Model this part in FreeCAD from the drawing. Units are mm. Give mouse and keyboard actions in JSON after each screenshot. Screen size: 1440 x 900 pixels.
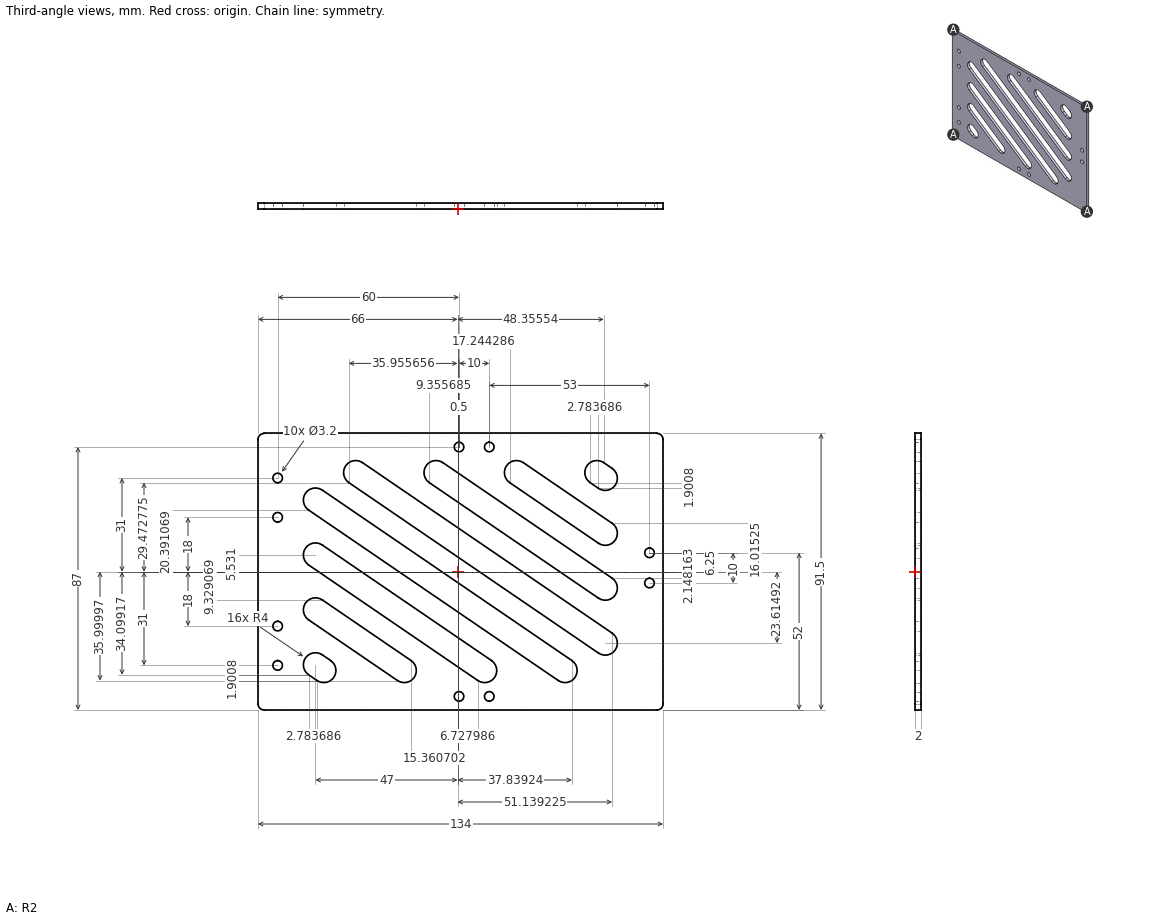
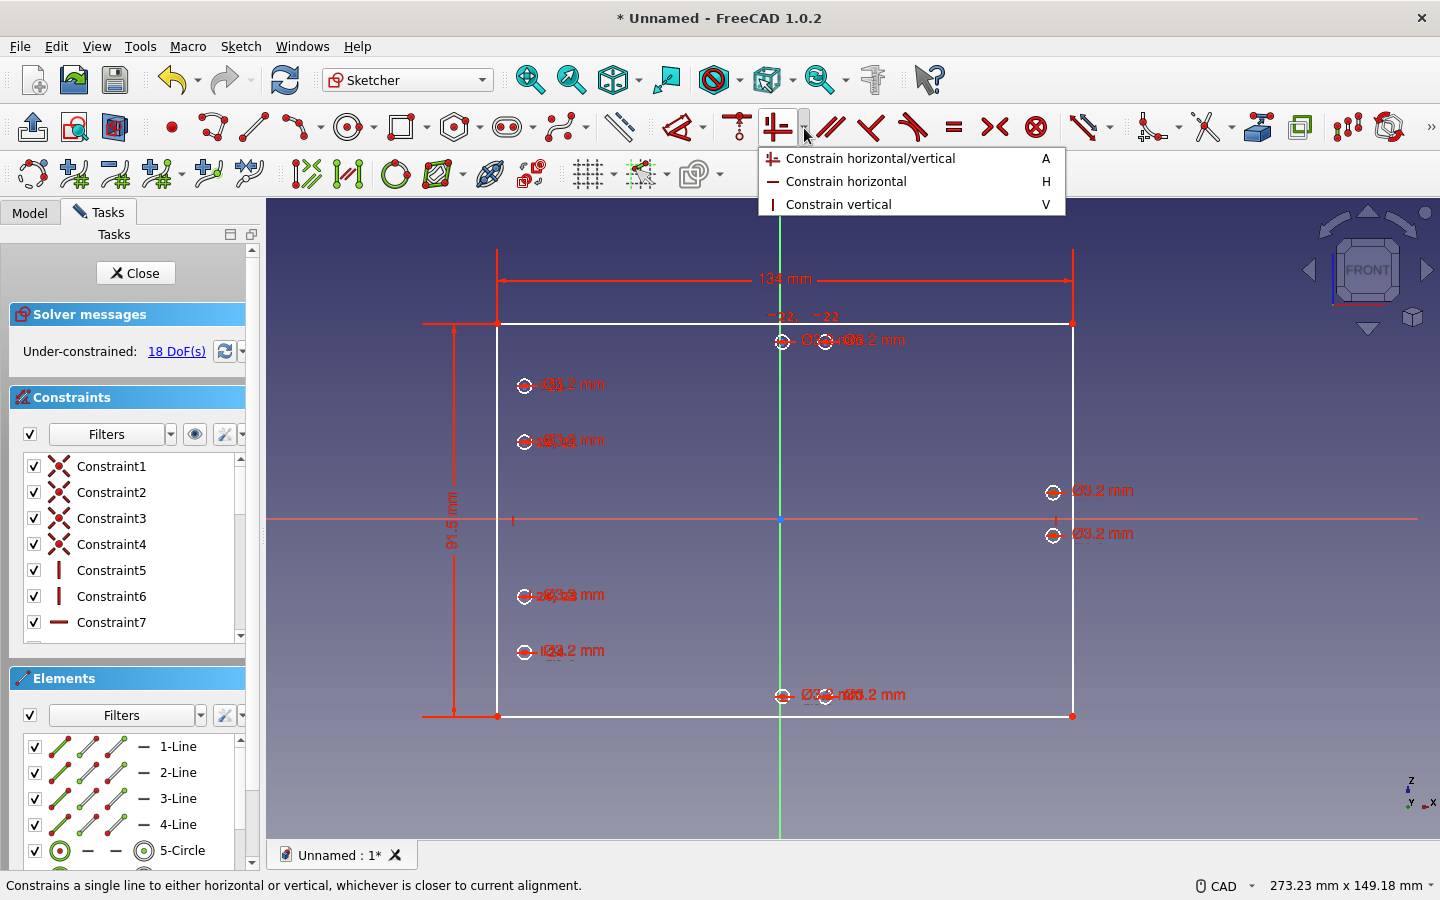
{"action": "left_click", "coordinate": [912, 204]}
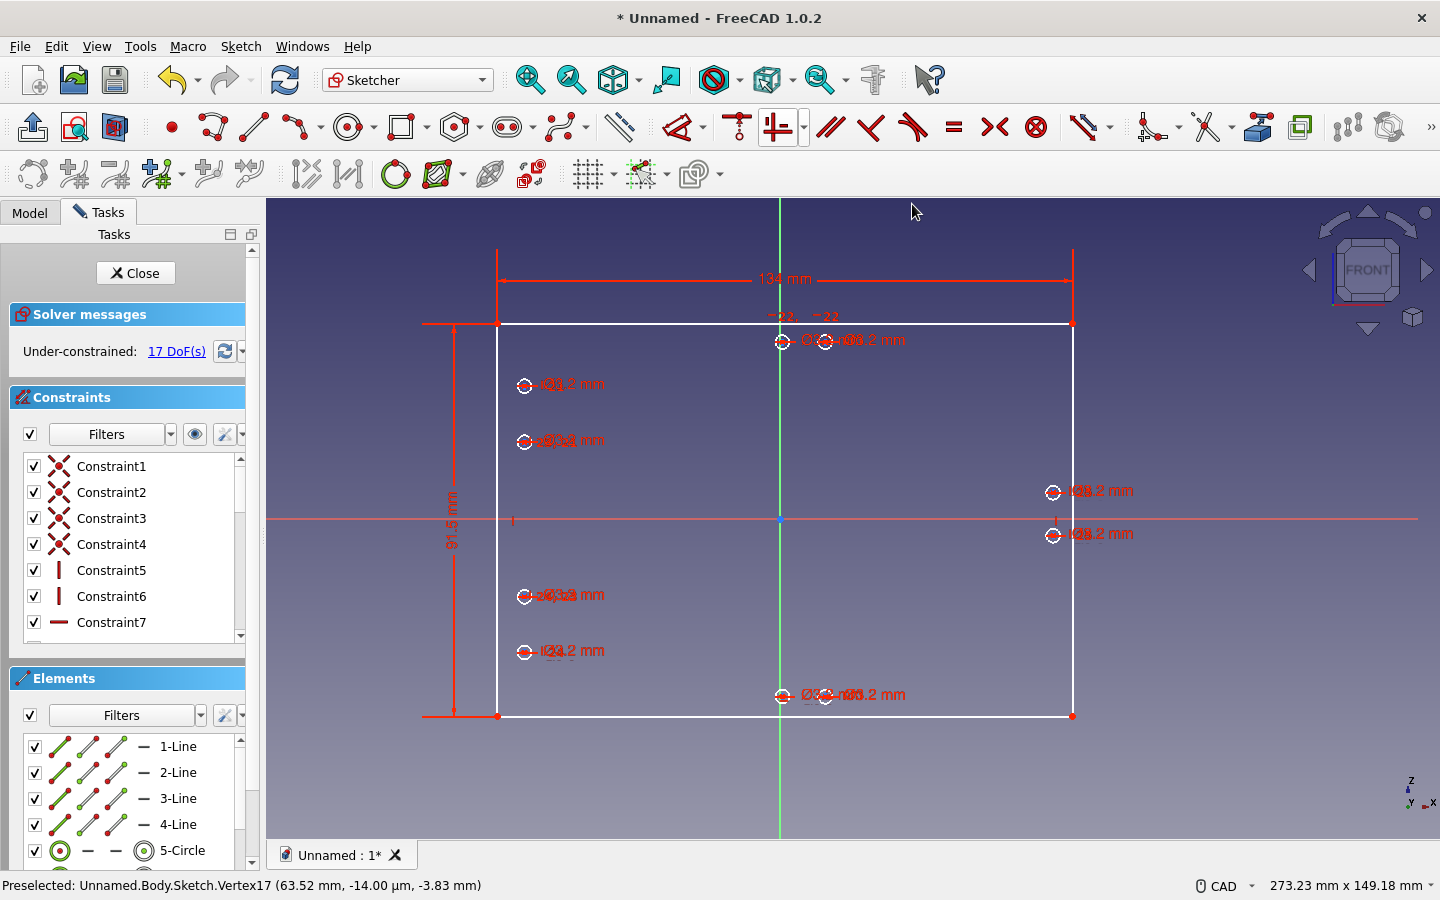
{"action": "left_click", "coordinate": [782, 697]}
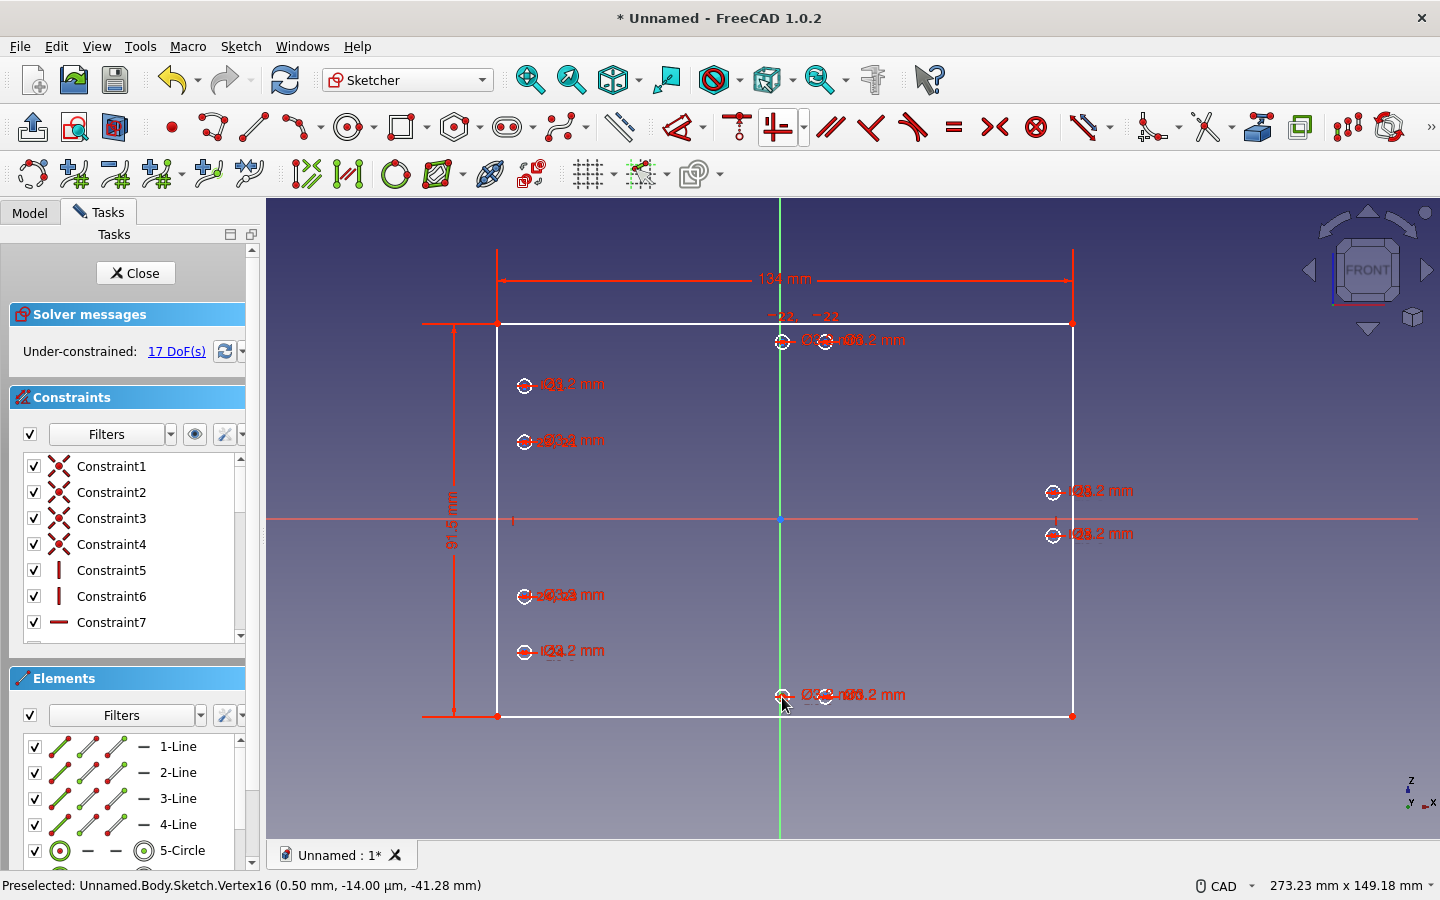
{"action": "left_click", "coordinate": [825, 697]}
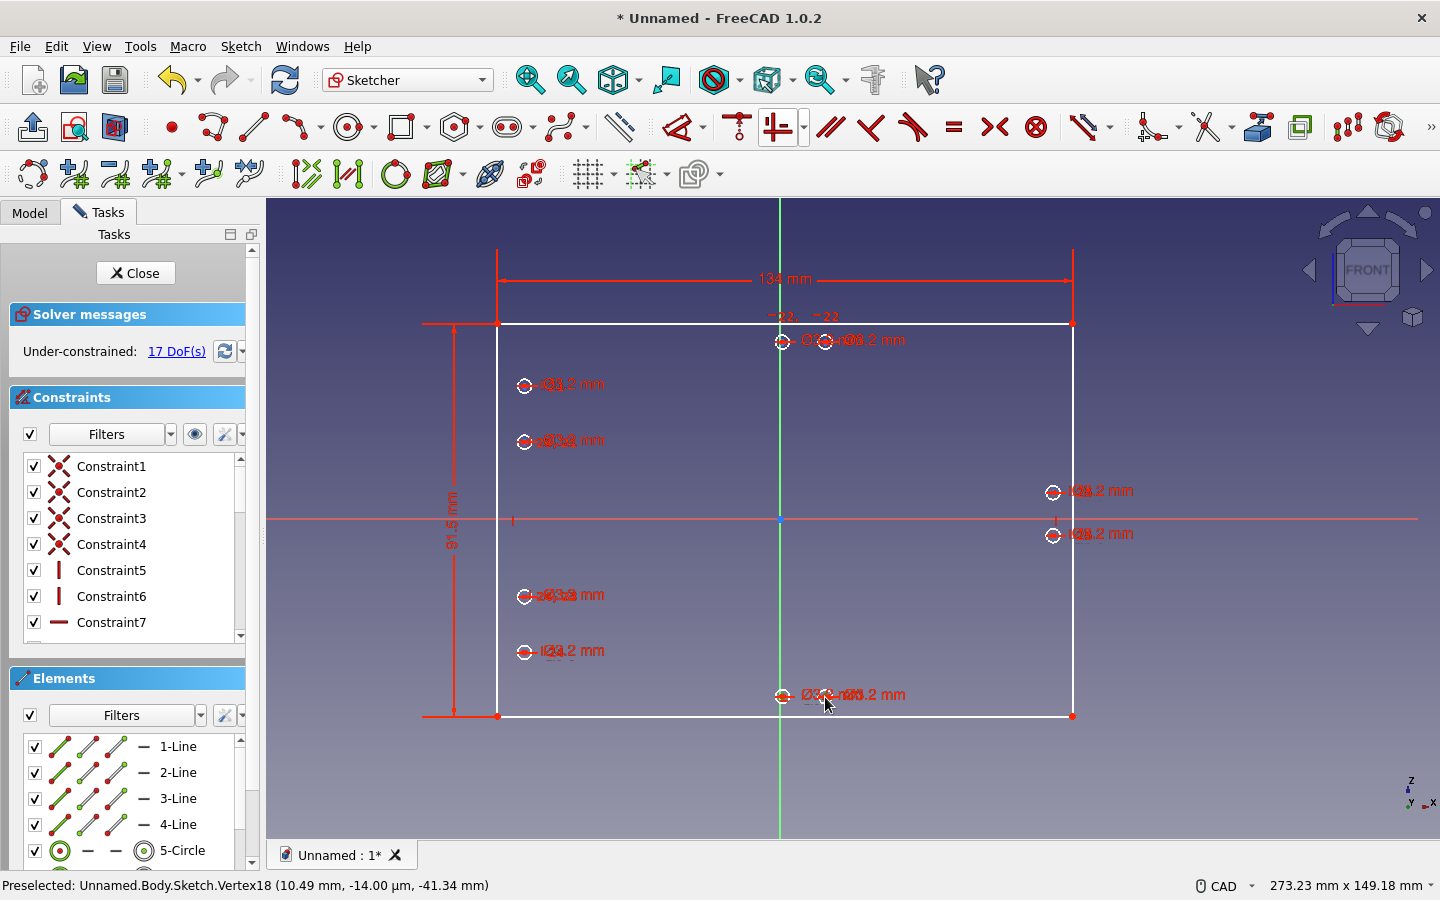
{"action": "left_click", "coordinate": [804, 128]}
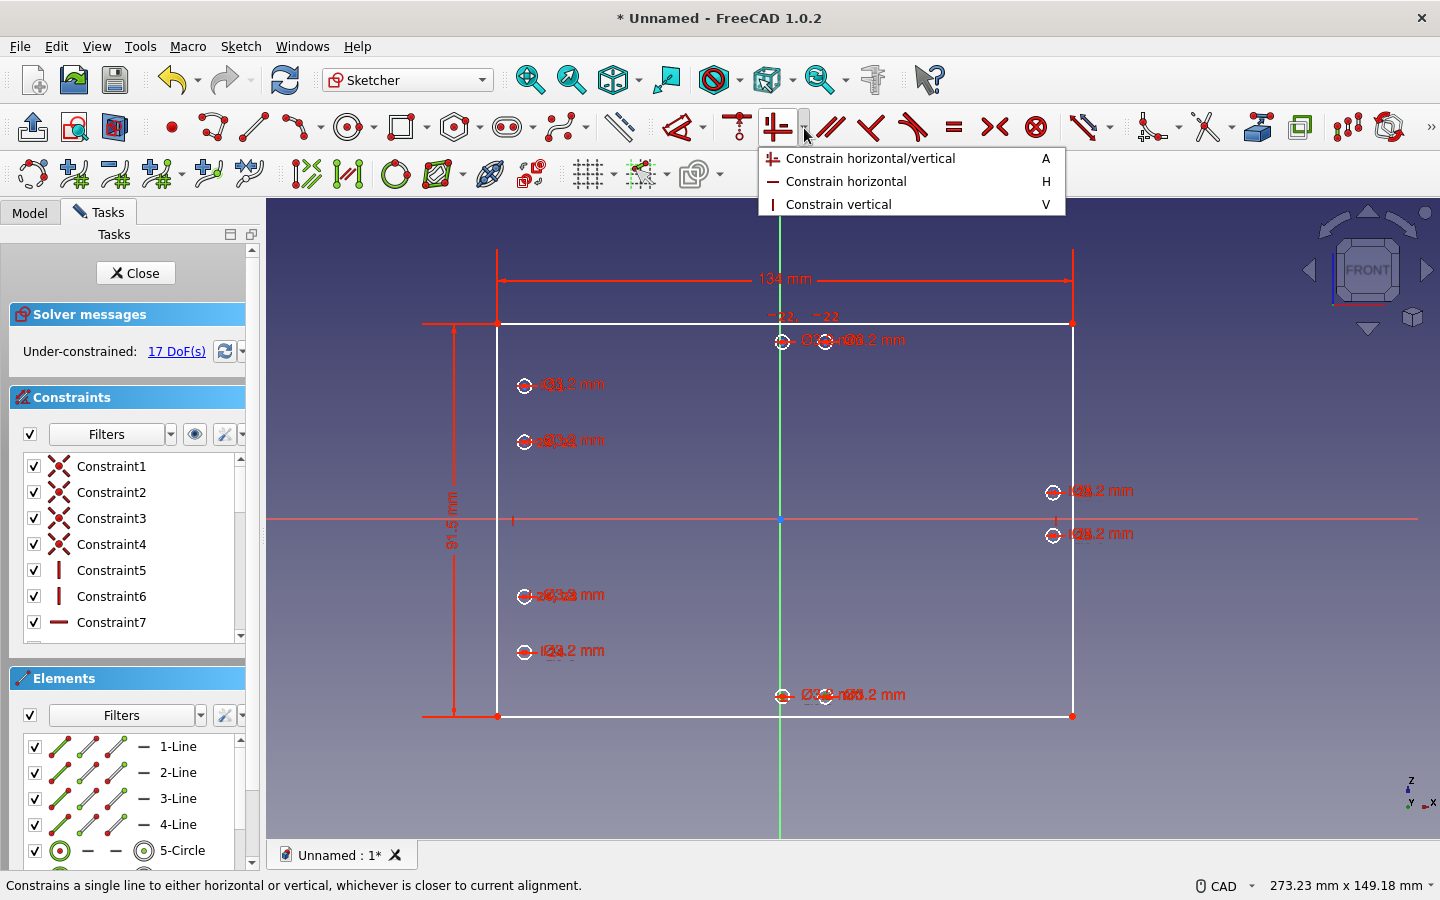
{"action": "left_click", "coordinate": [912, 182]}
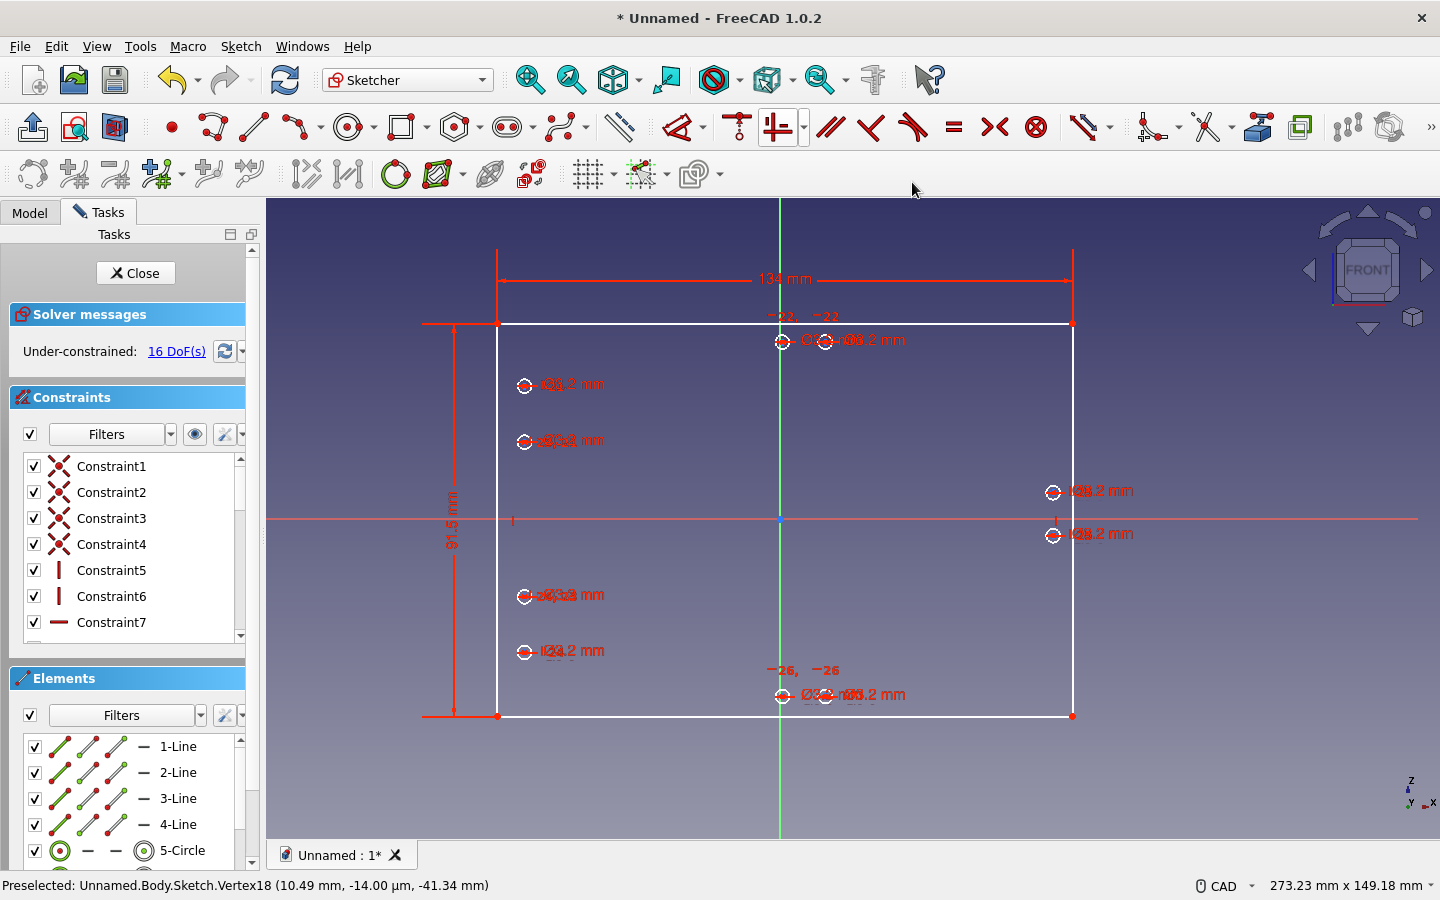
{"action": "left_click", "coordinate": [782, 342]}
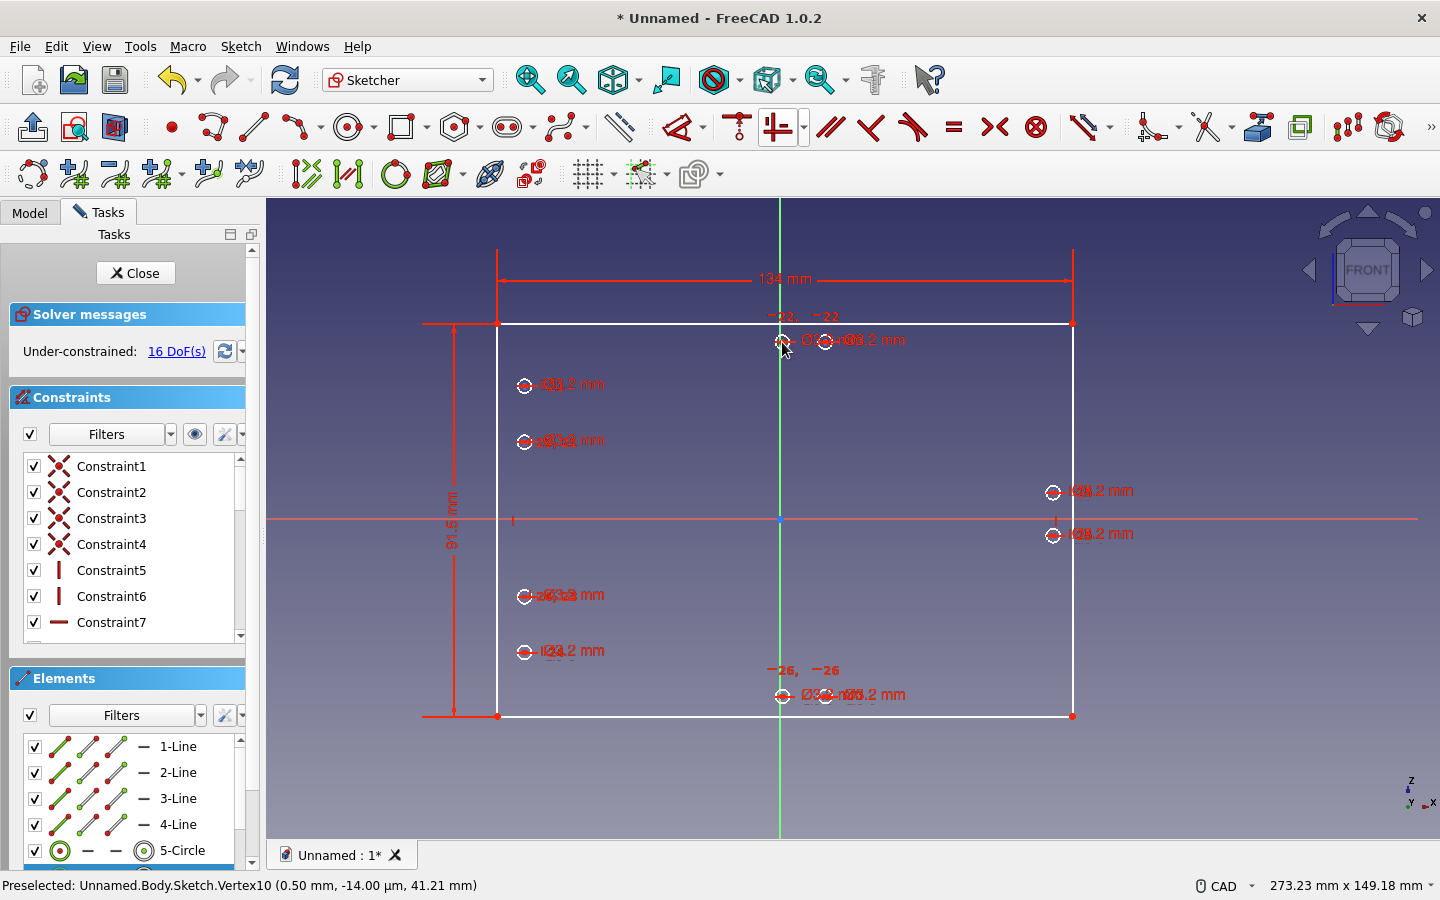
{"action": "left_click", "coordinate": [782, 697]}